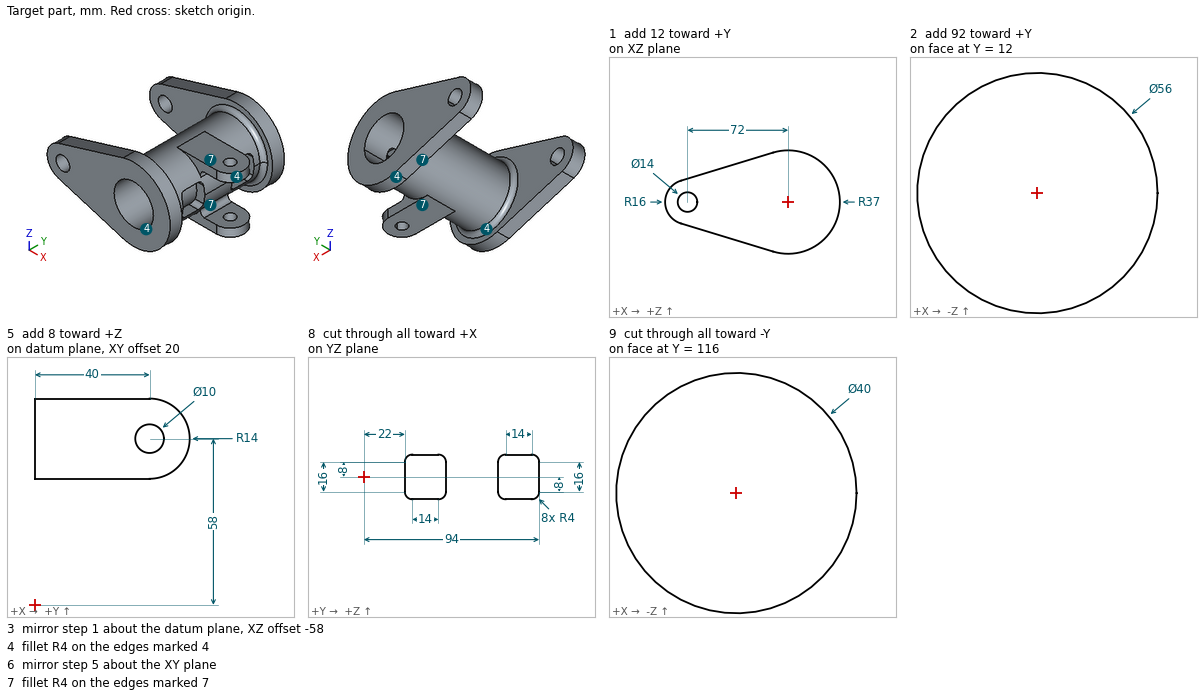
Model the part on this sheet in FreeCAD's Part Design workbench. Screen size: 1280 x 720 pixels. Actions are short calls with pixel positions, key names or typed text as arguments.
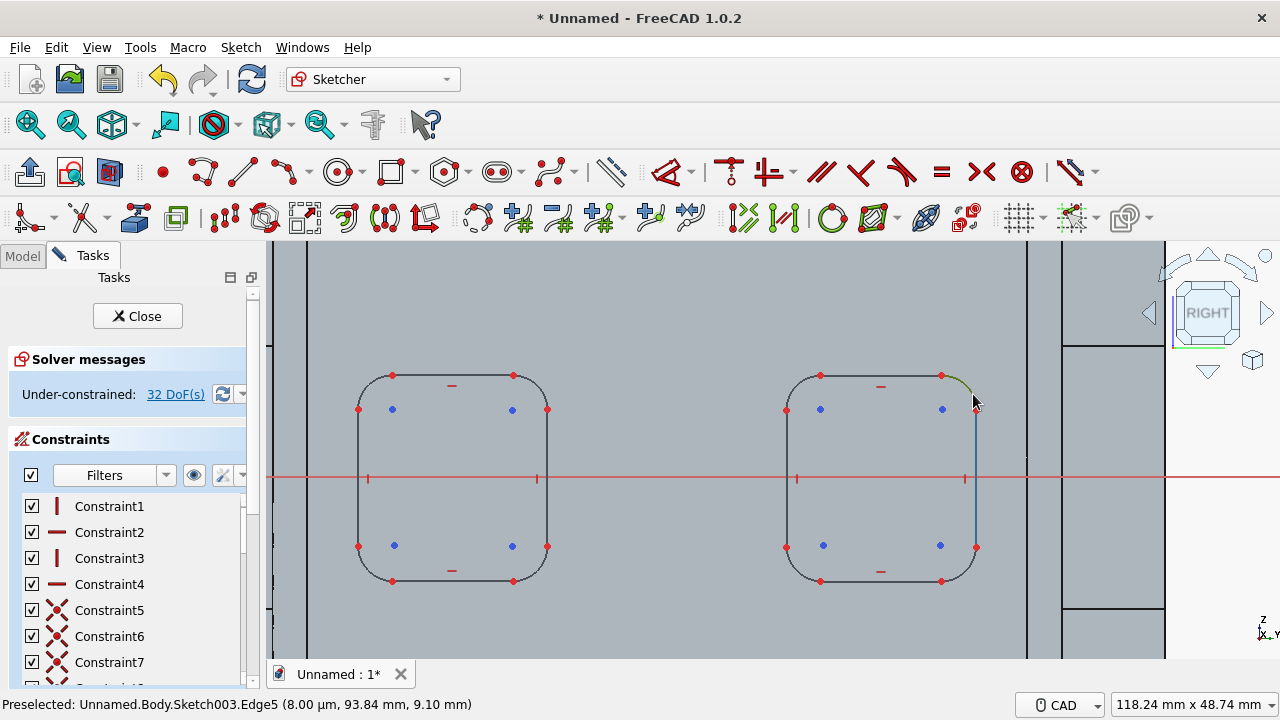
click(902, 172)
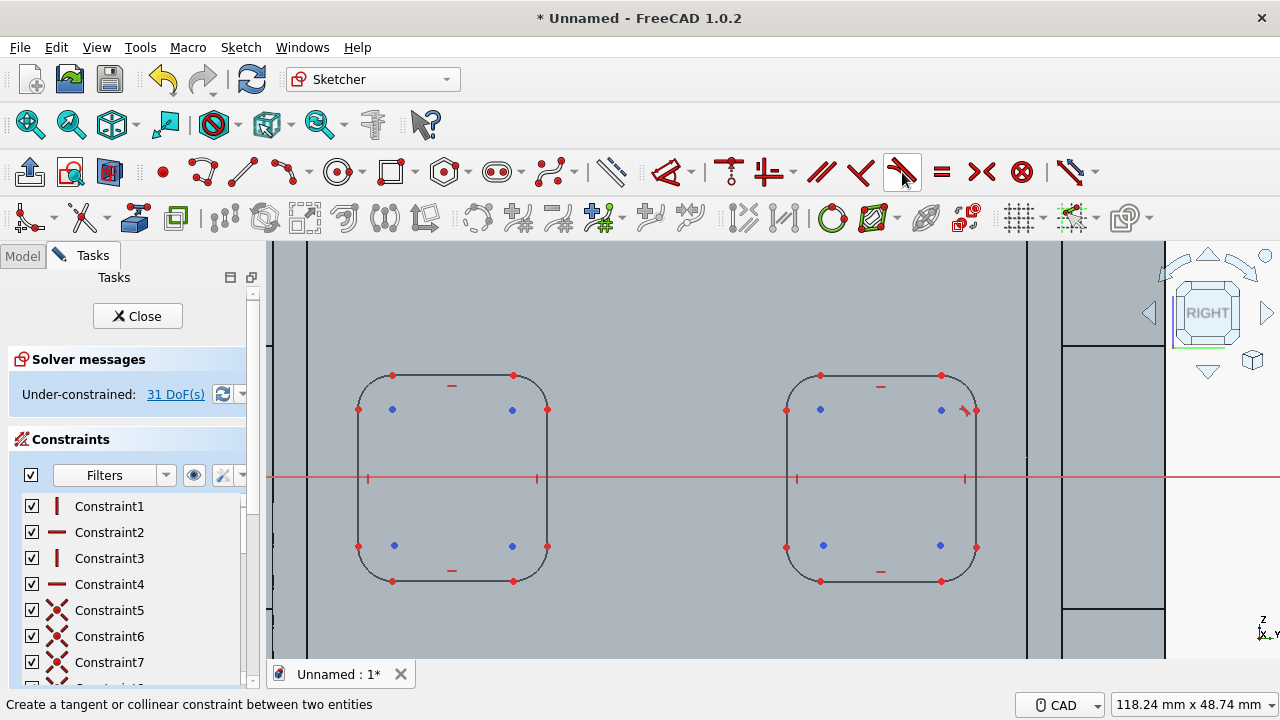
click(976, 506)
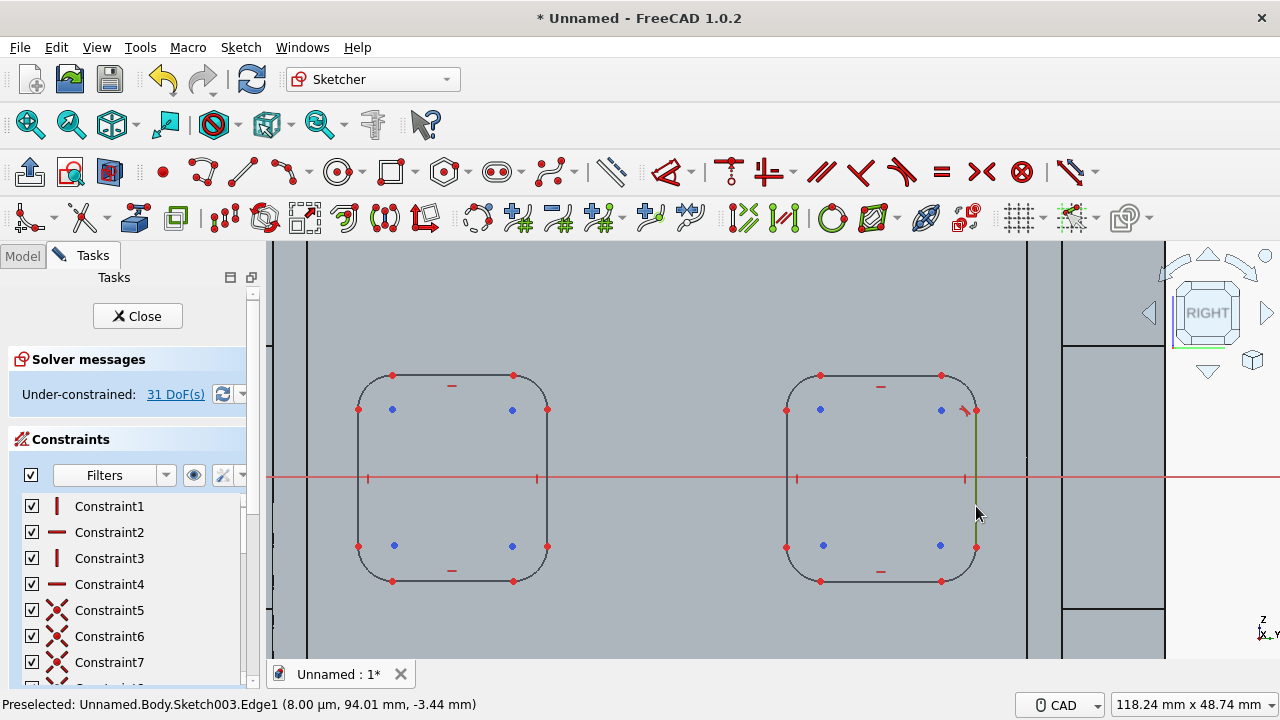
click(957, 578)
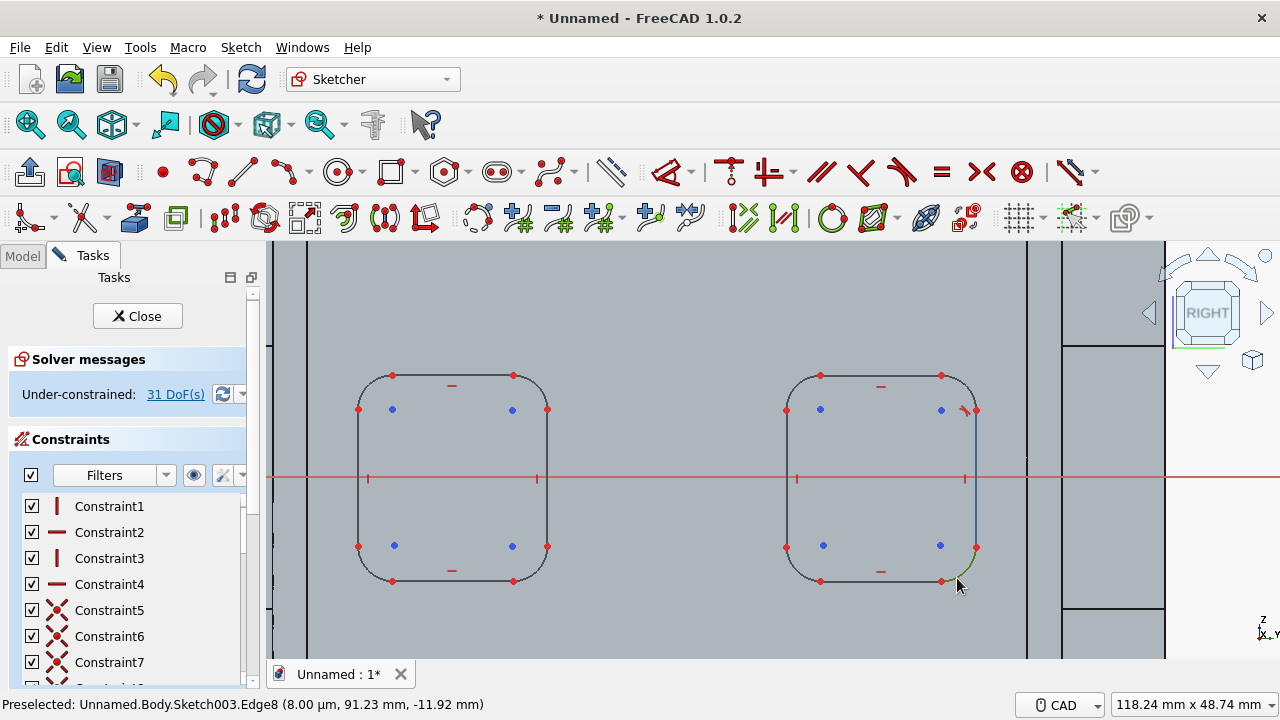
click(902, 172)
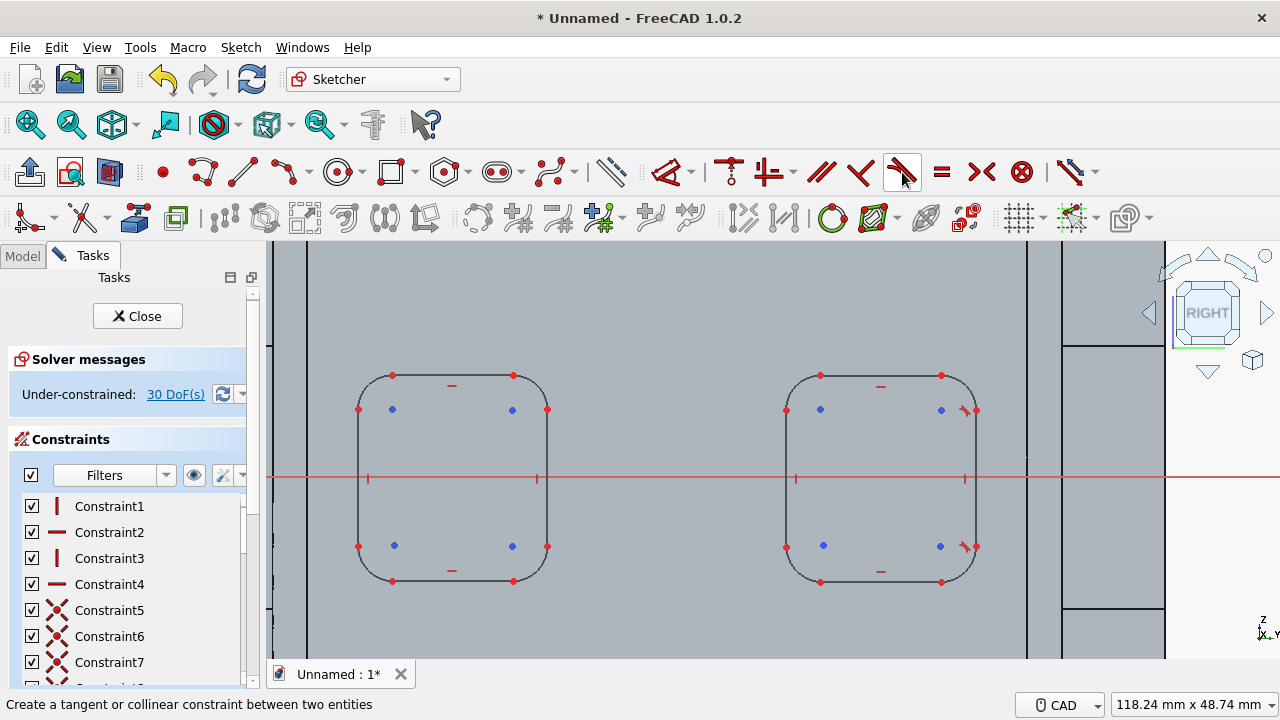
click(905, 376)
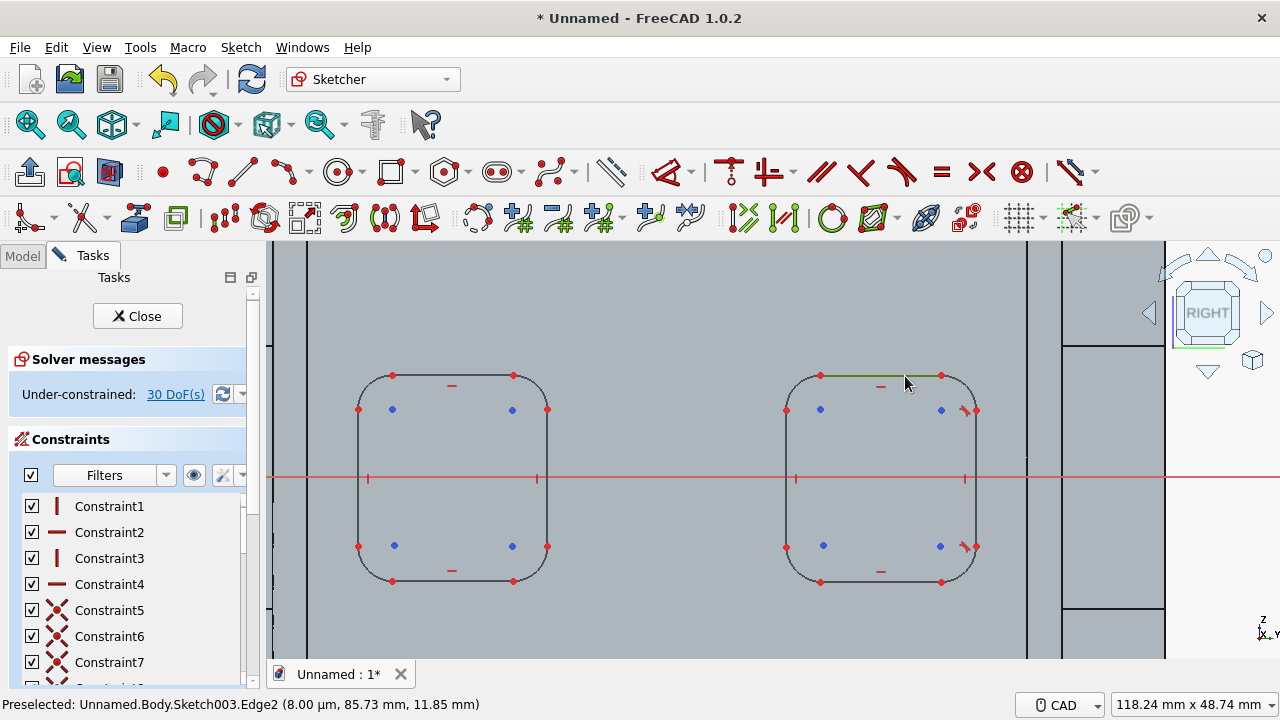
click(972, 395)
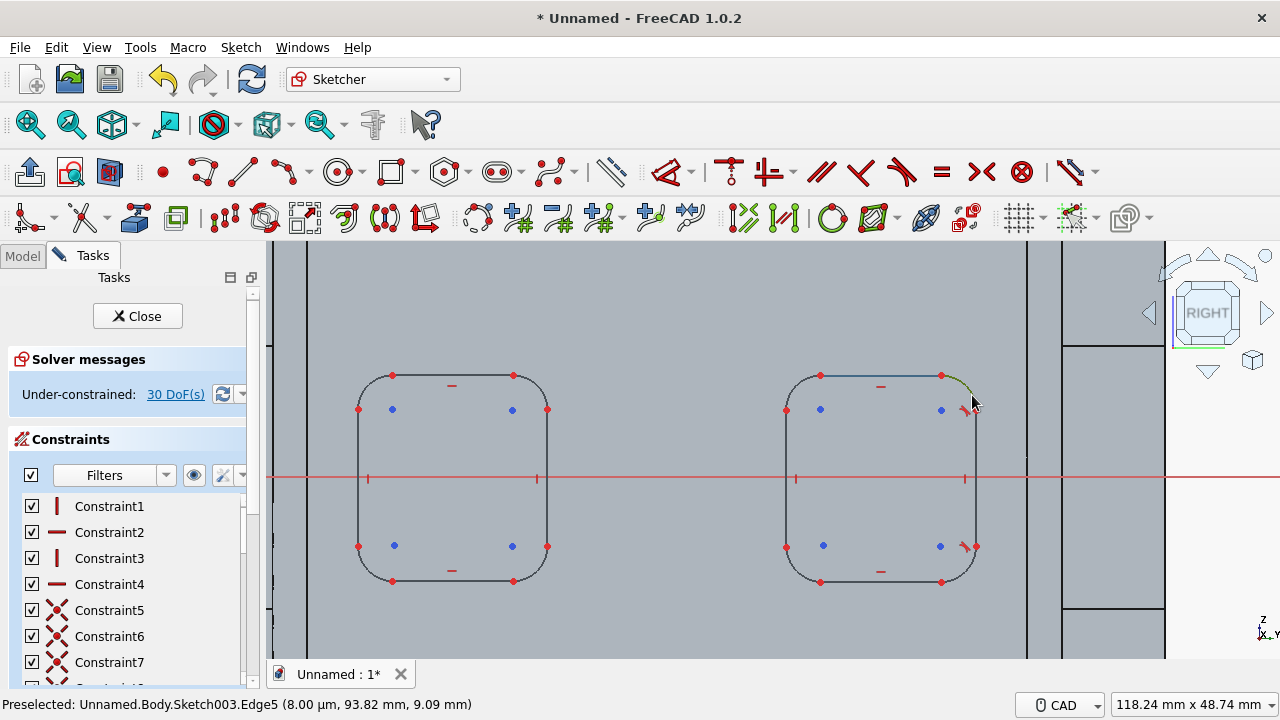
click(902, 172)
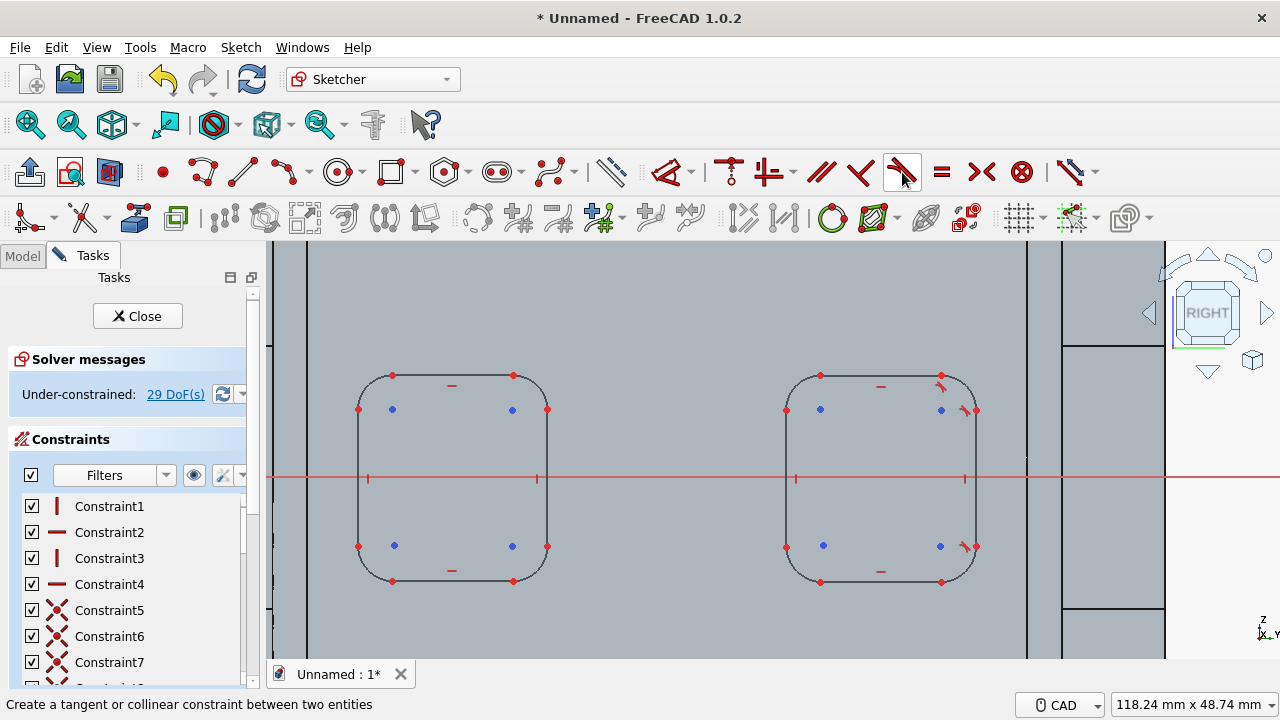
click(905, 376)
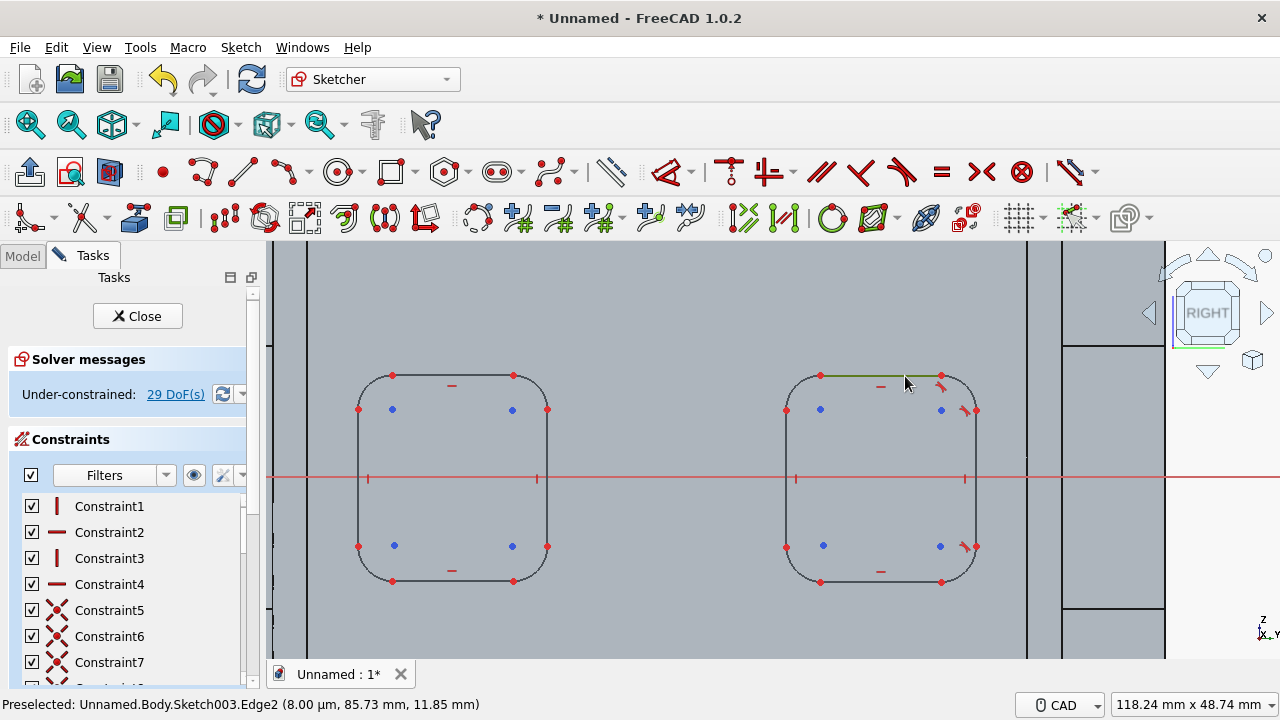
click(805, 379)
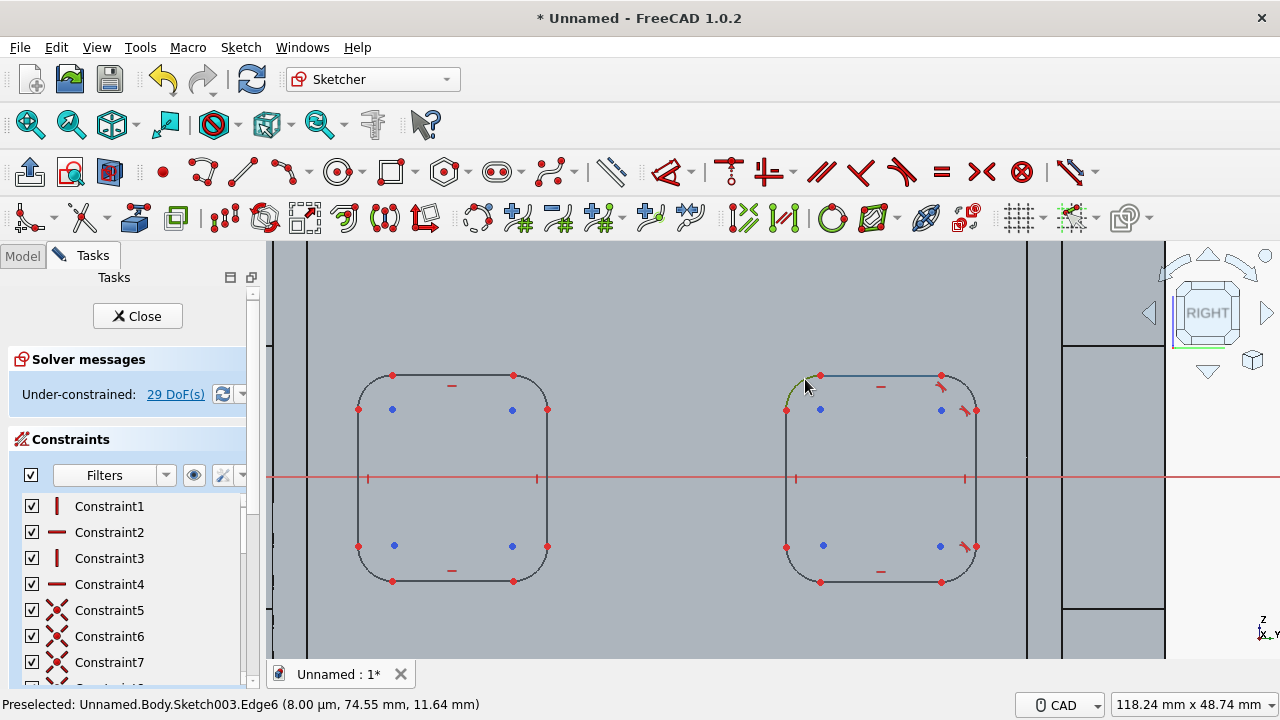
key(t)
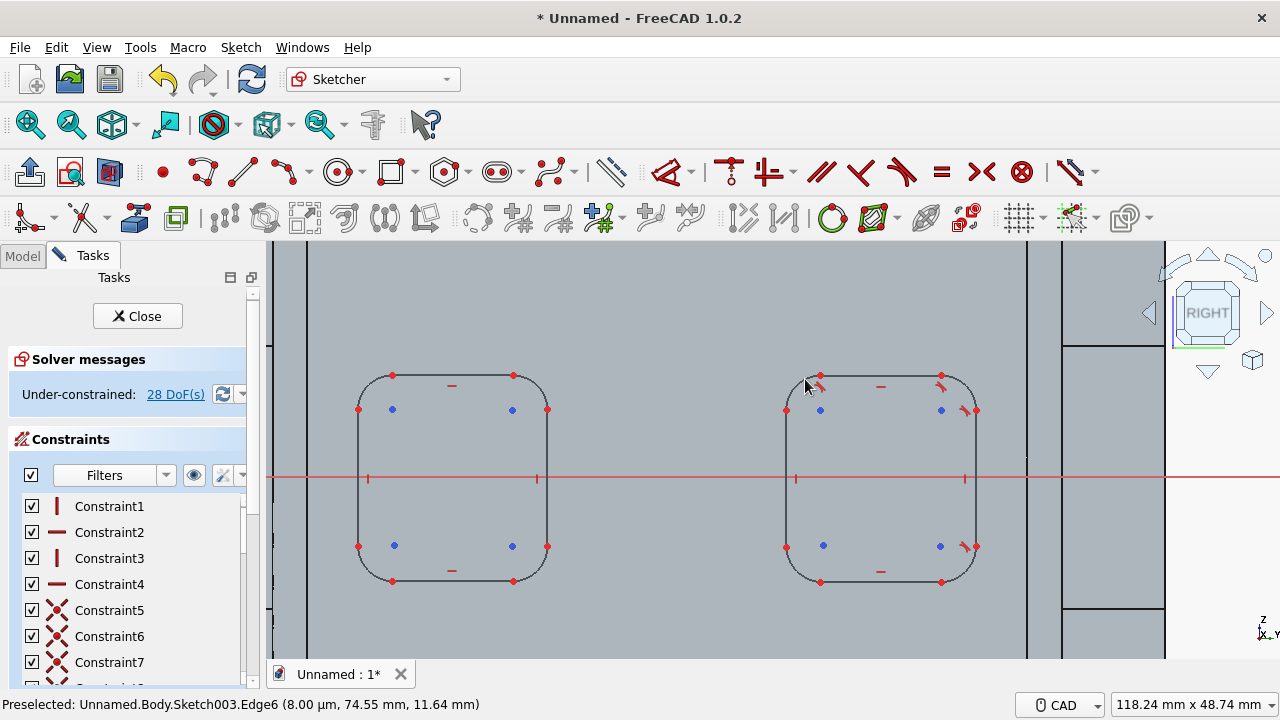
click(786, 451)